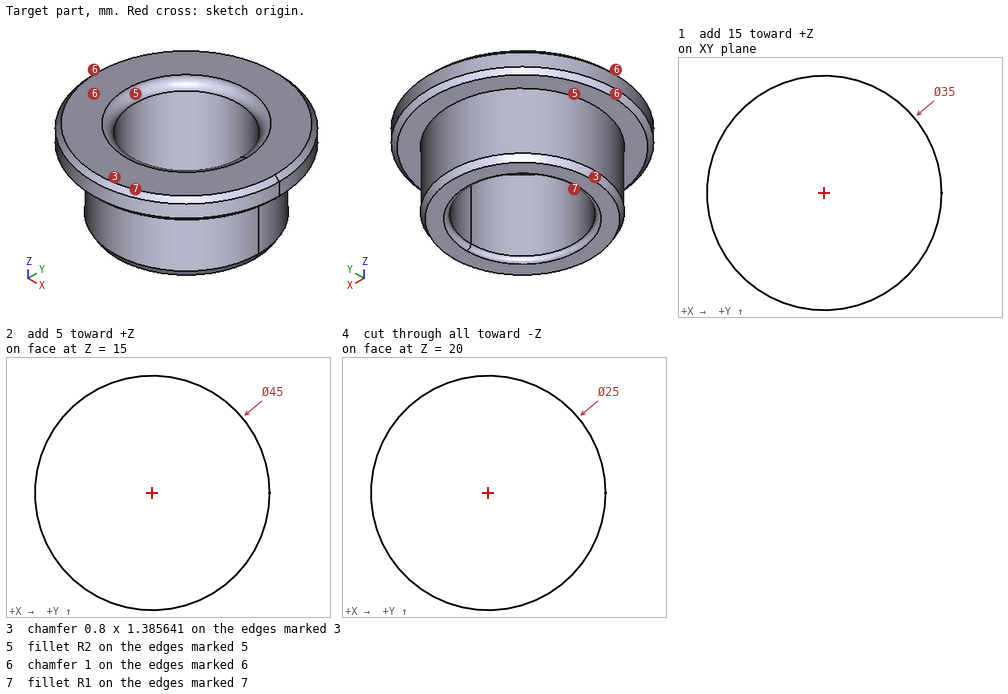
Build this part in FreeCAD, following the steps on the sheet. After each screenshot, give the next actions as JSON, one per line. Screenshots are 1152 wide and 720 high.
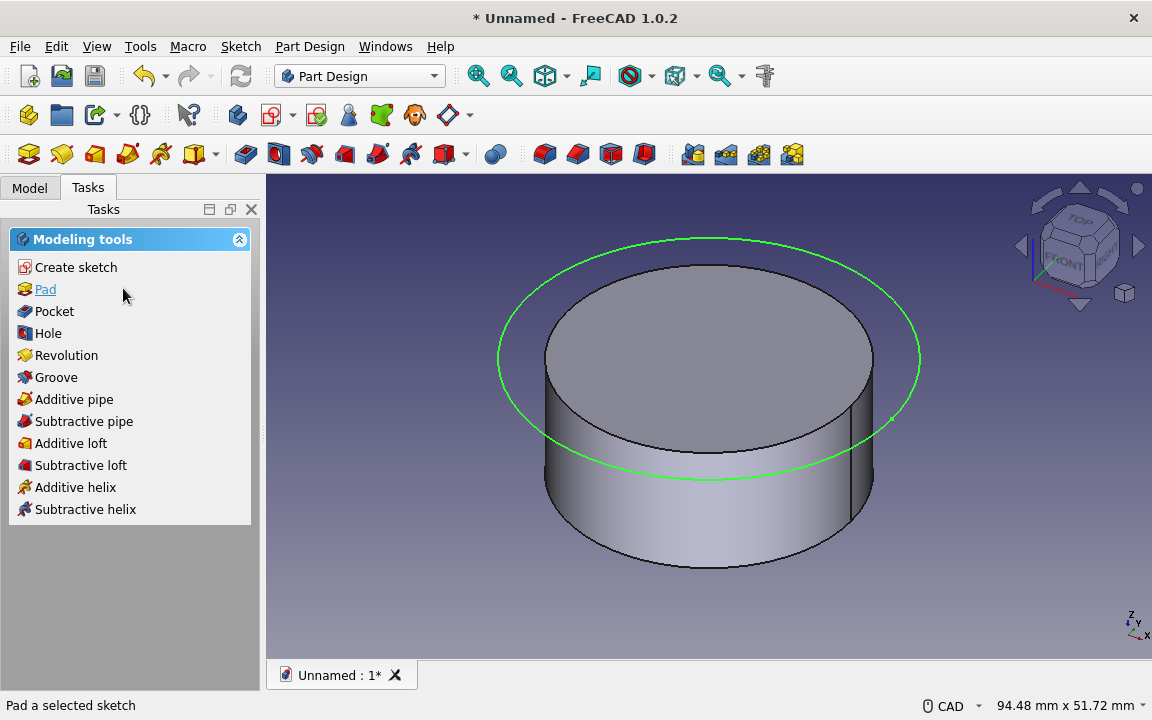
{"action": "left_click", "coordinate": [29, 154]}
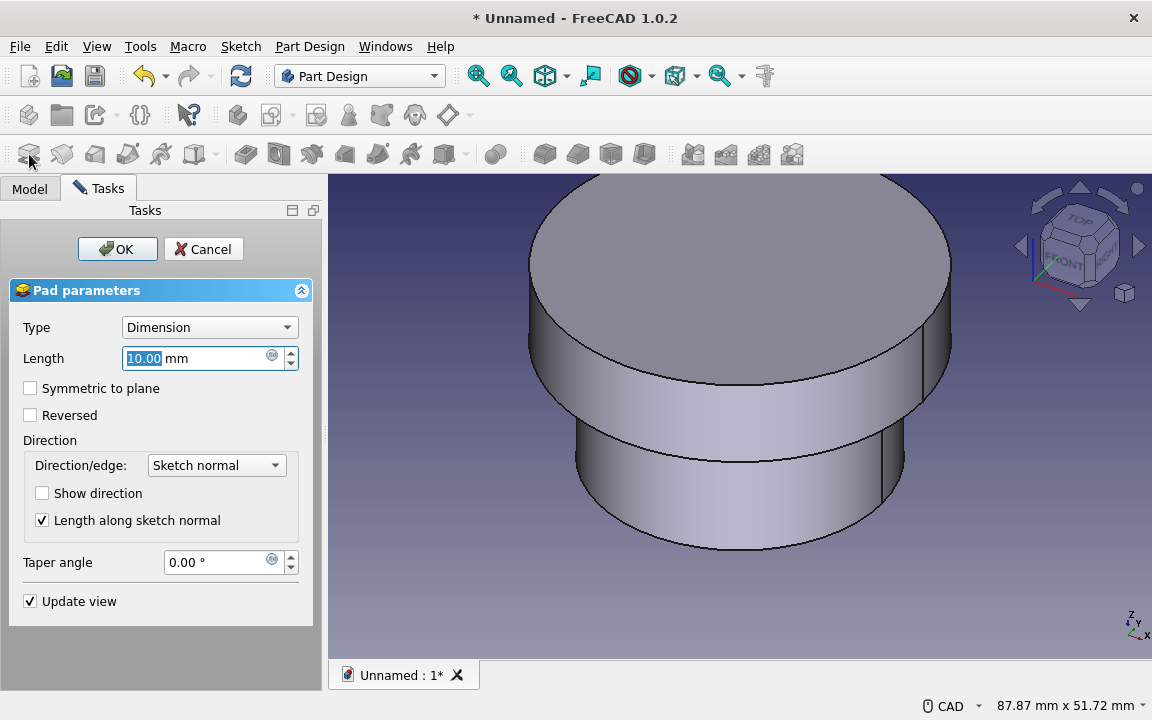
{"action": "type", "text": "5"}
{"action": "key", "text": "Tab"}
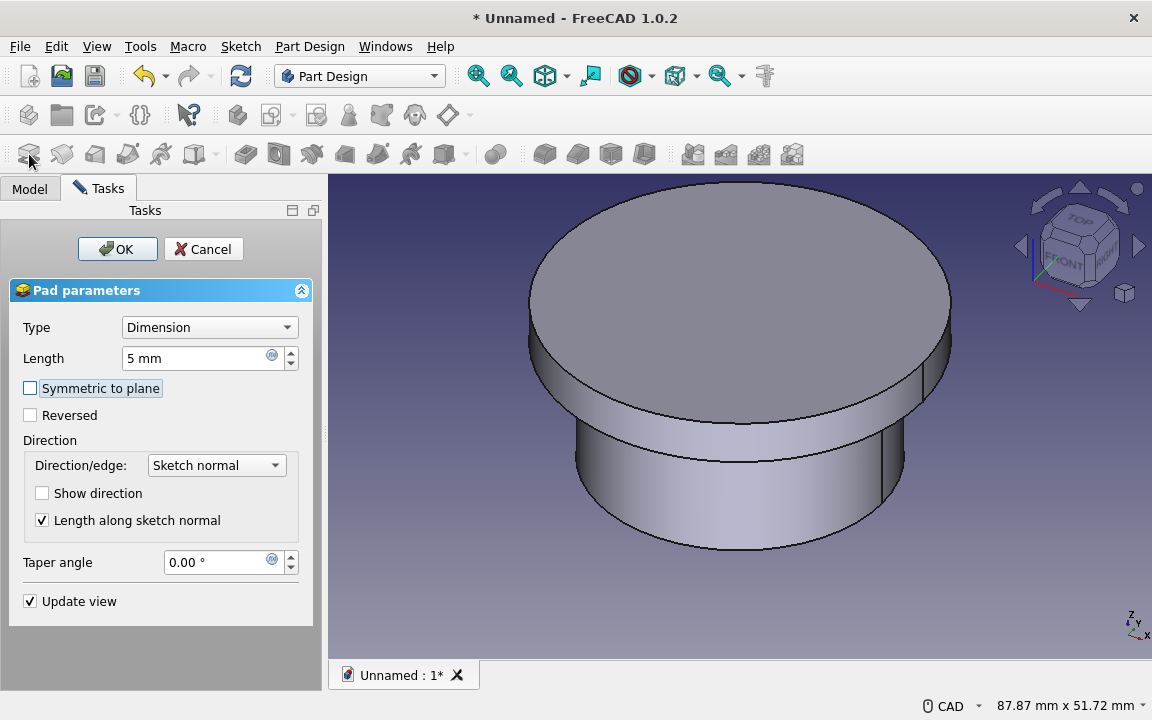
{"action": "left_click", "coordinate": [118, 249]}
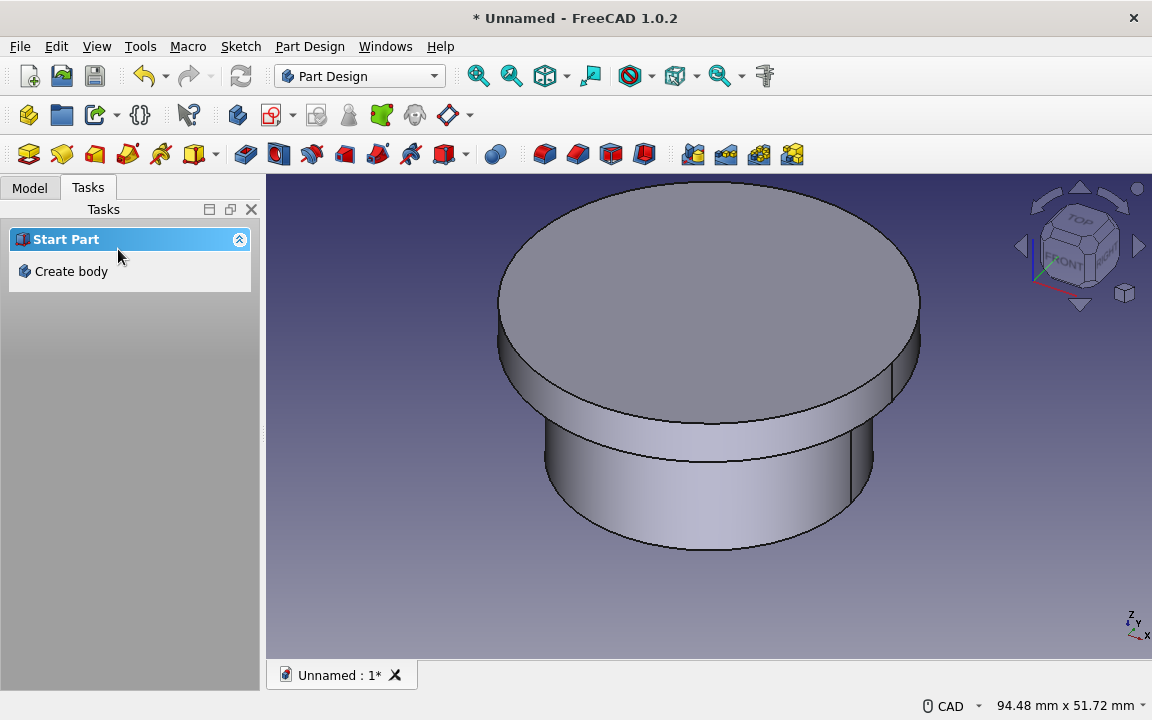
{"action": "key", "text": "v f"}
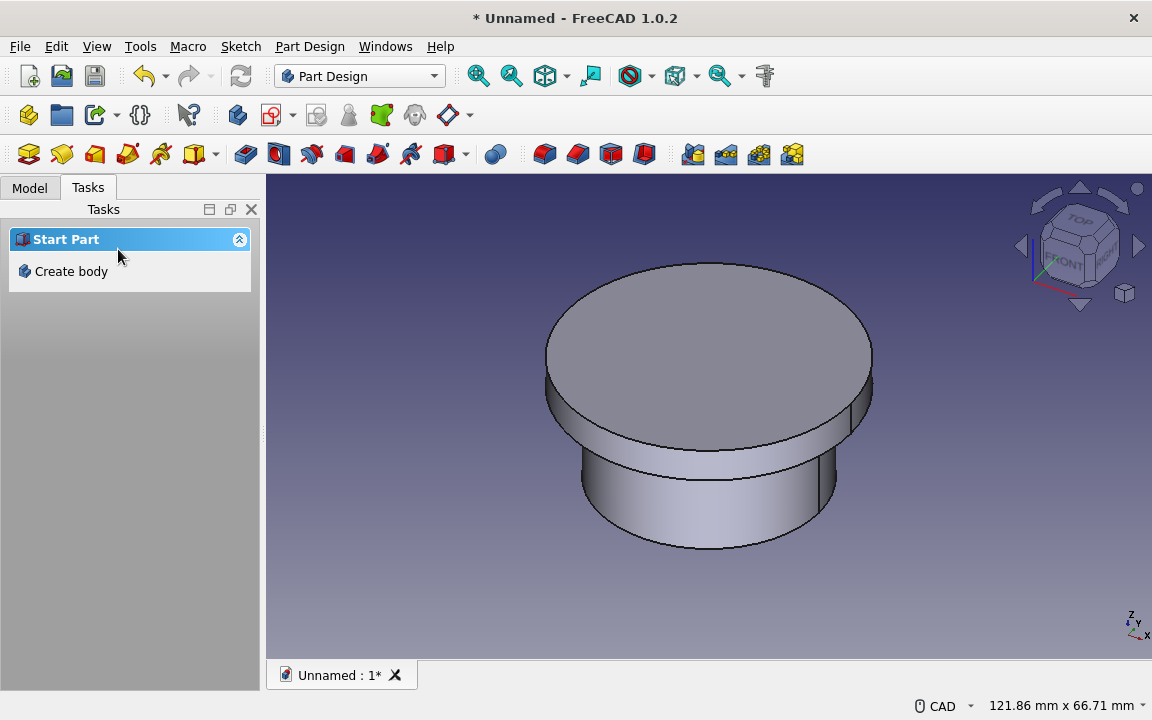
{"action": "key", "text": "0"}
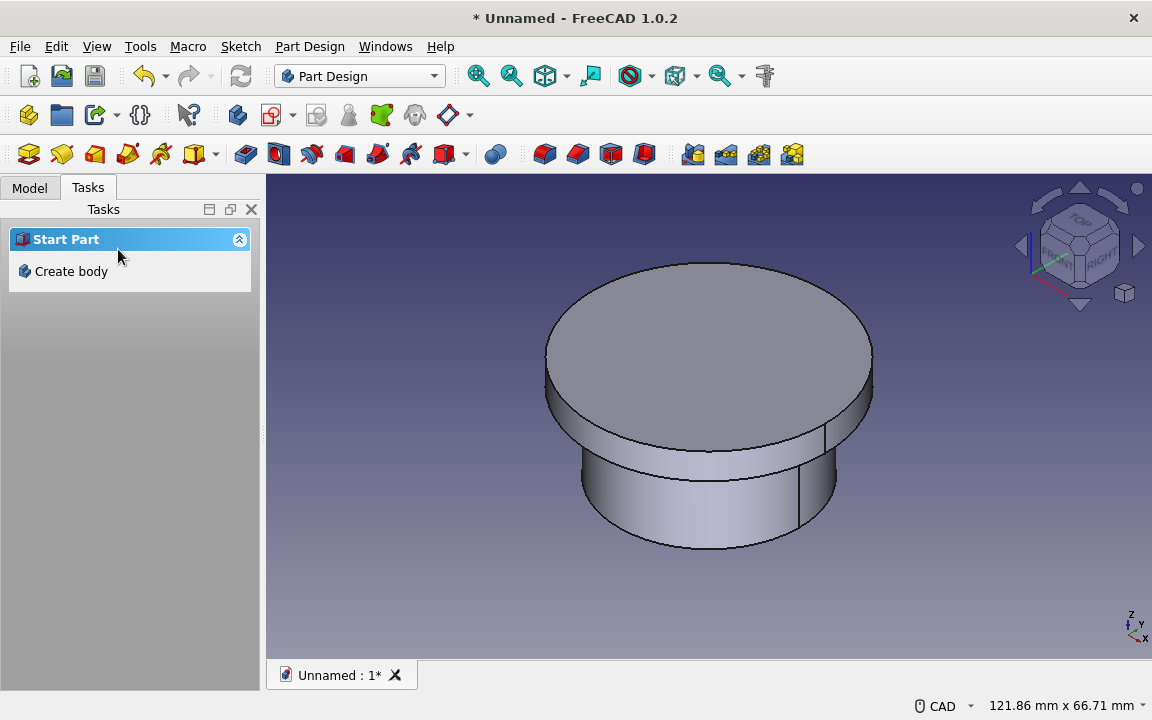
{"action": "key", "text": "2"}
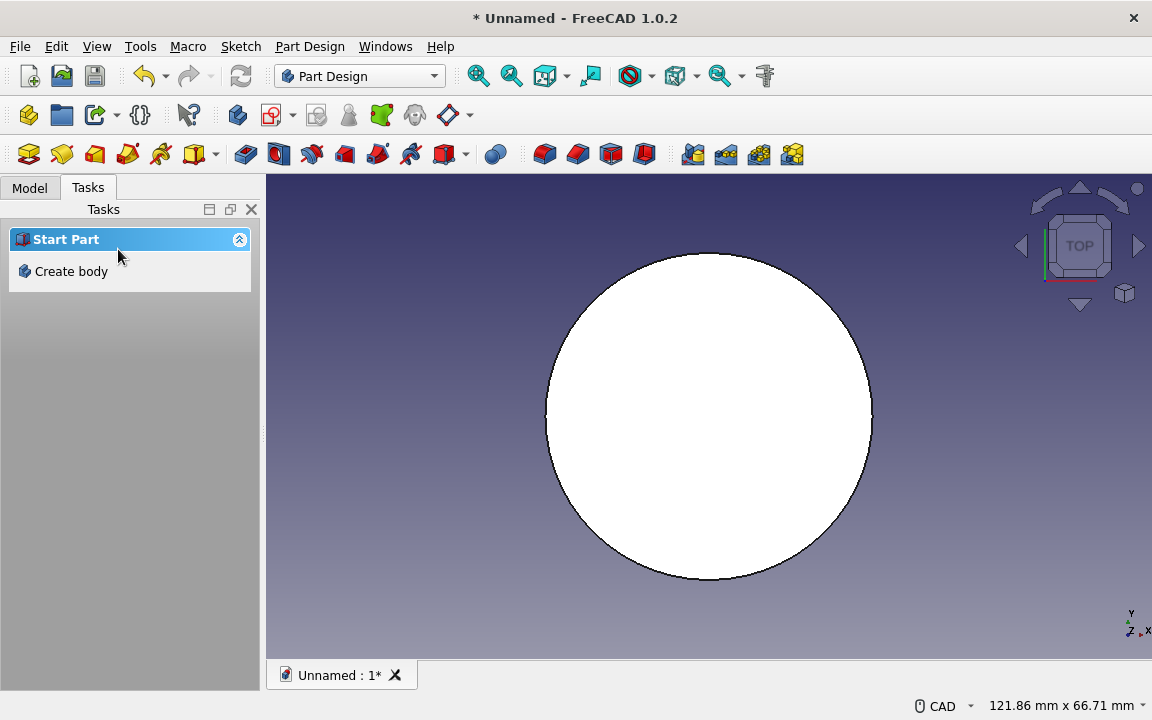
{"action": "key", "text": "1"}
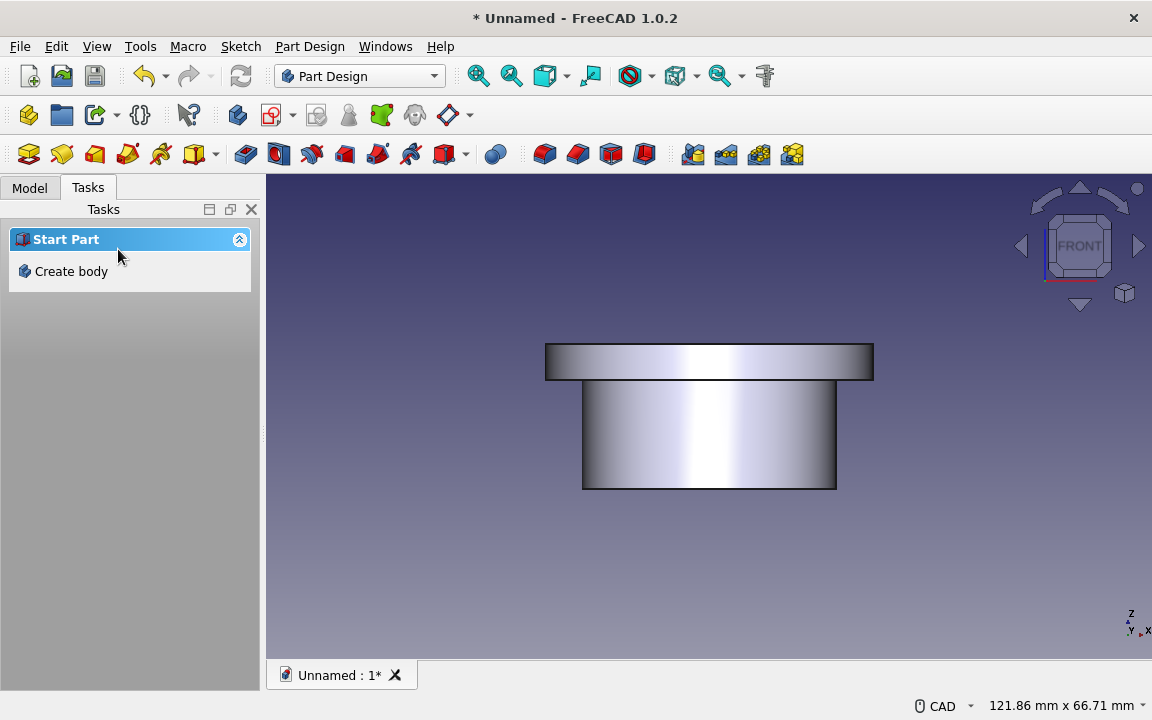
{"action": "left_click", "coordinate": [479, 76]}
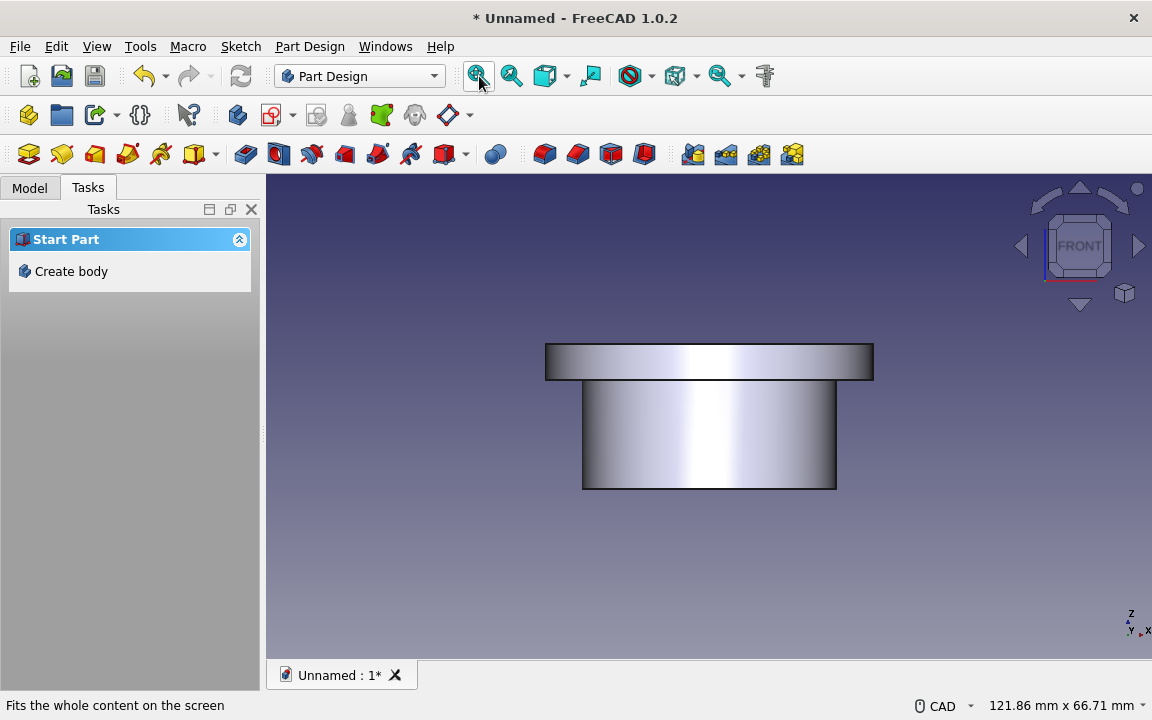
{"action": "left_click", "coordinate": [606, 488]}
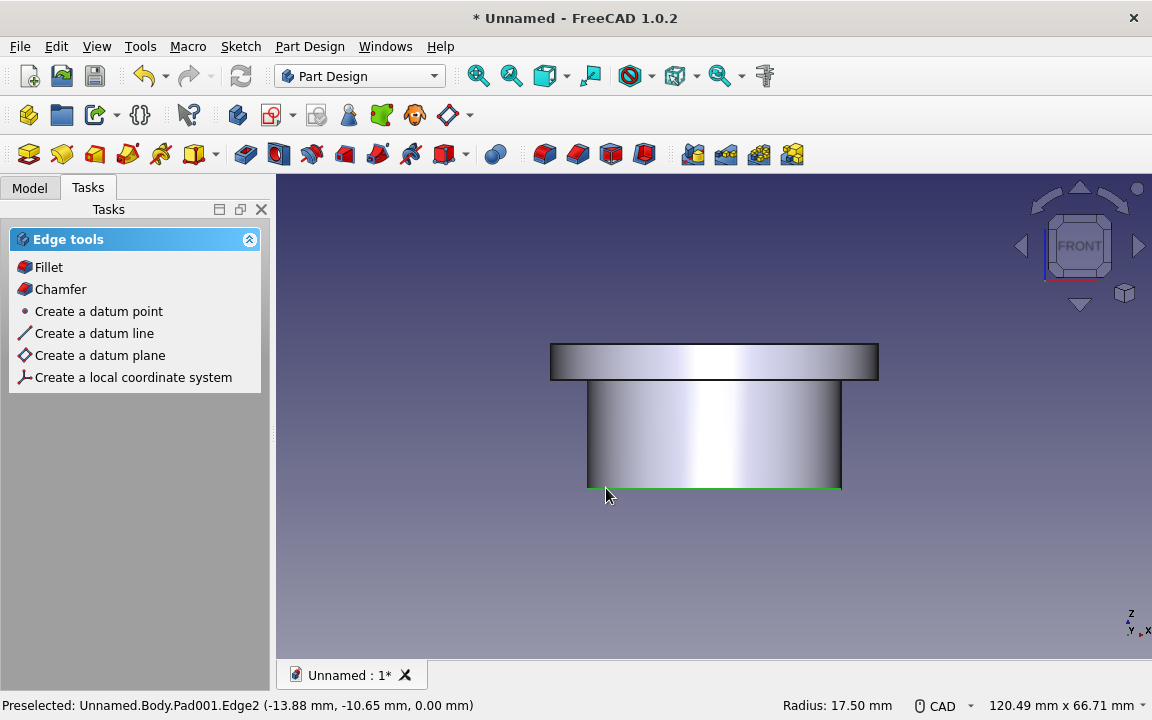
{"action": "left_click", "coordinate": [578, 154]}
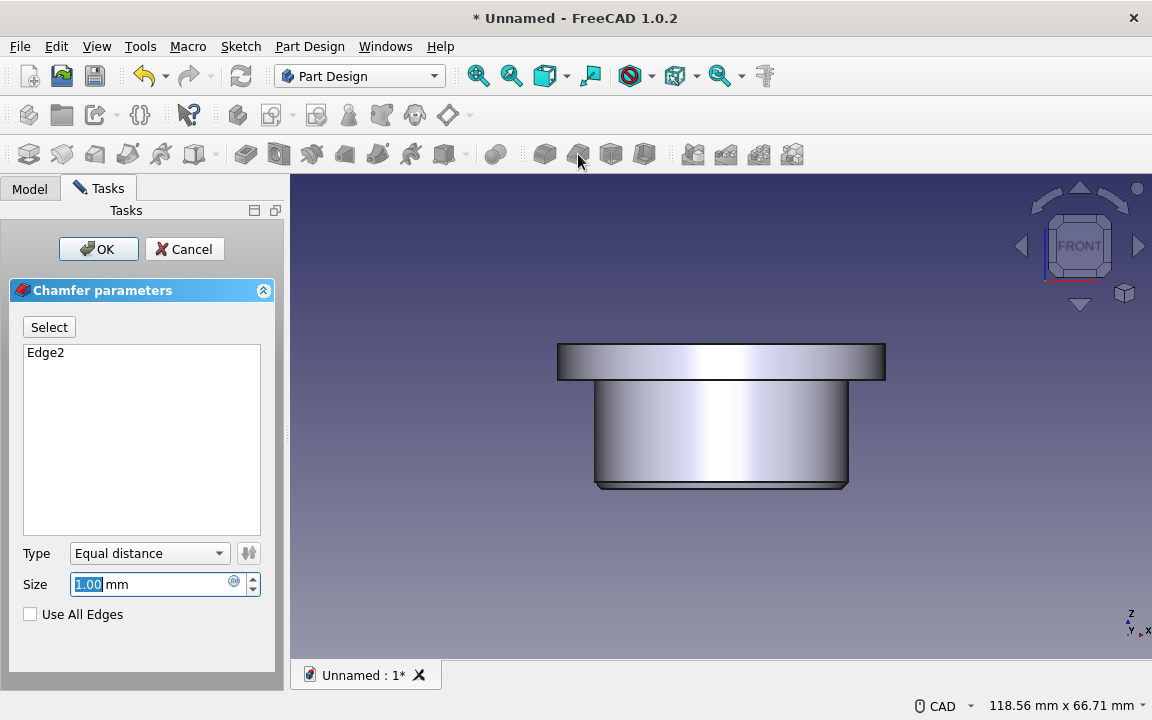
{"action": "type", "text": "0.8"}
{"action": "key", "text": "Tab"}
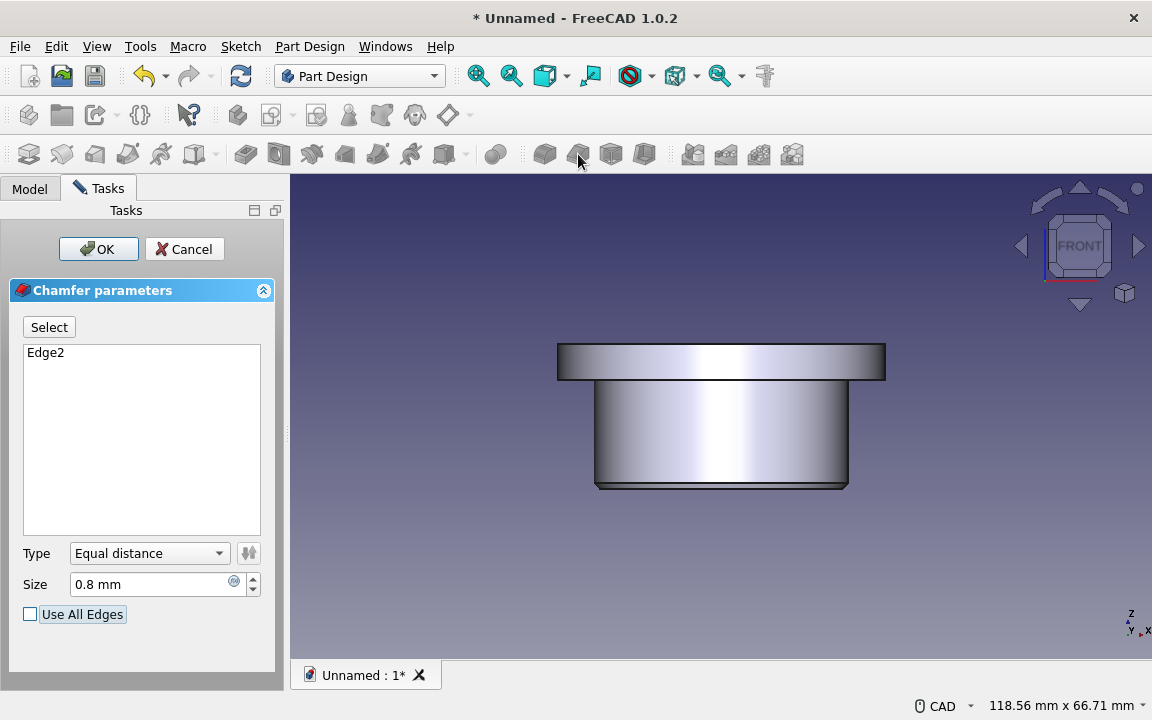
{"action": "left_click", "coordinate": [150, 554]}